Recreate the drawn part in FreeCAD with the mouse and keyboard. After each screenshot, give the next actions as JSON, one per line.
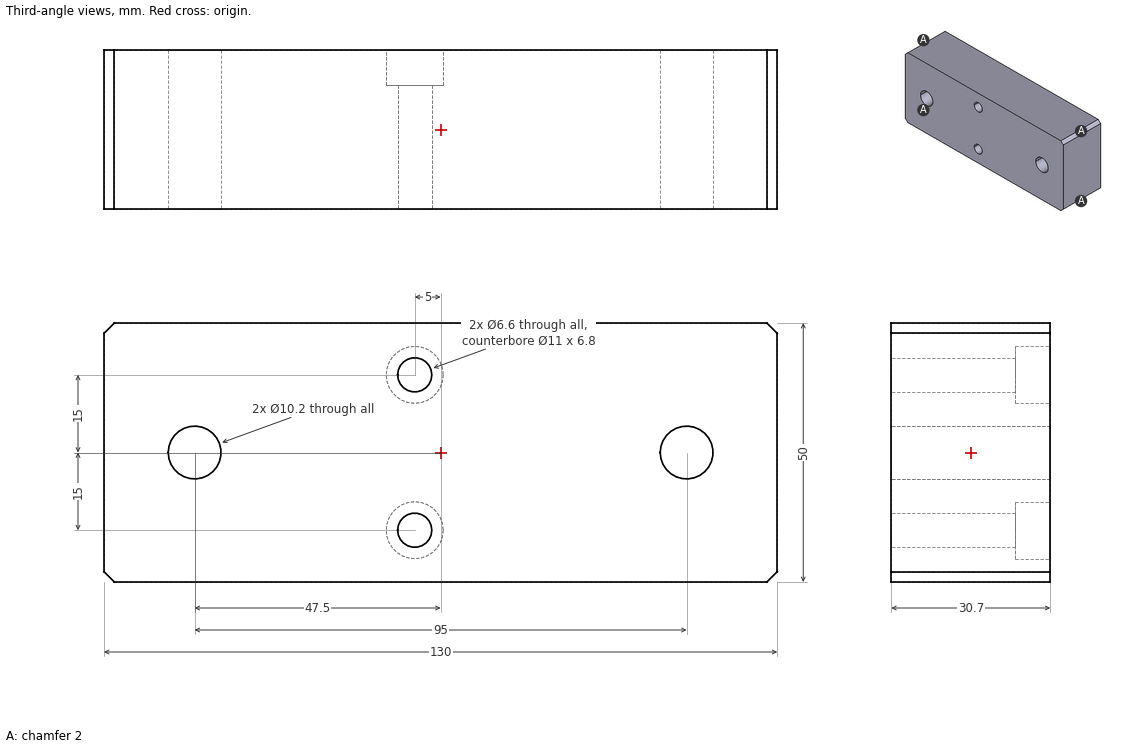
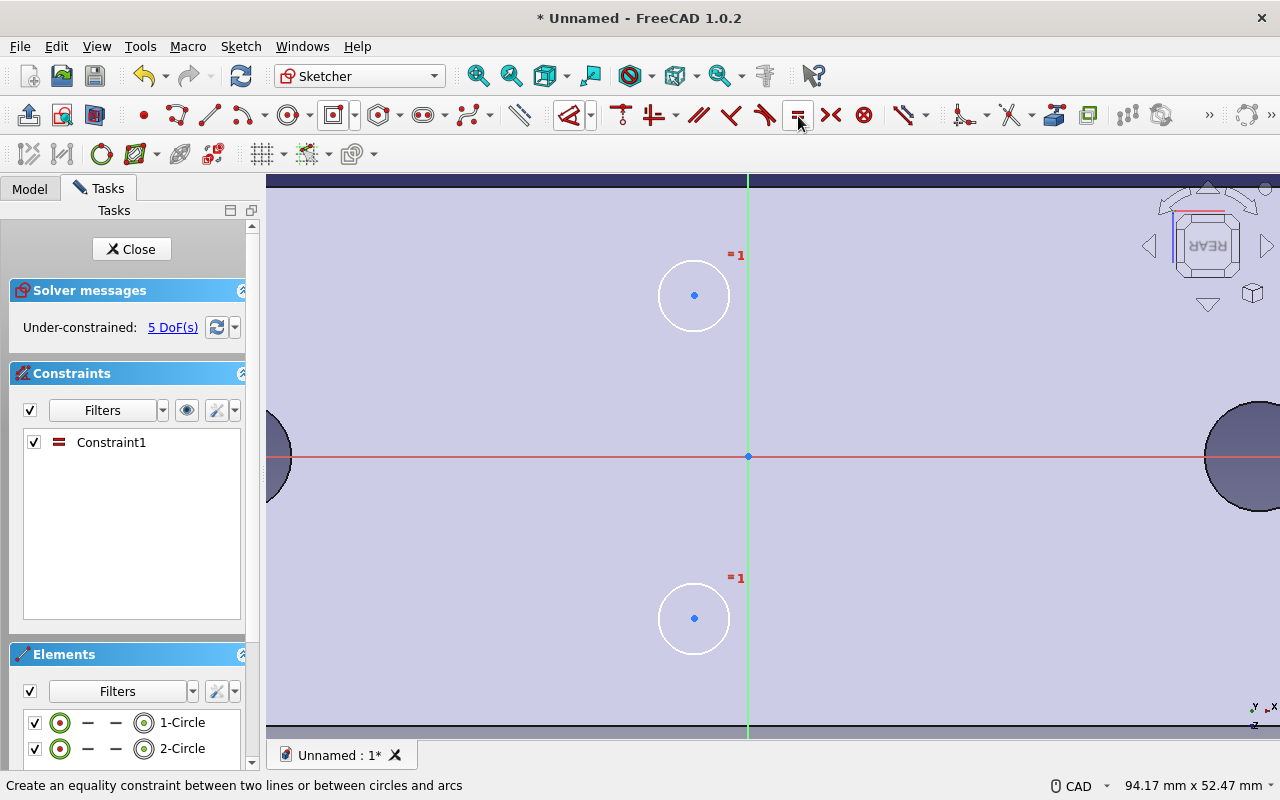
{"action": "left_click", "coordinate": [694, 619]}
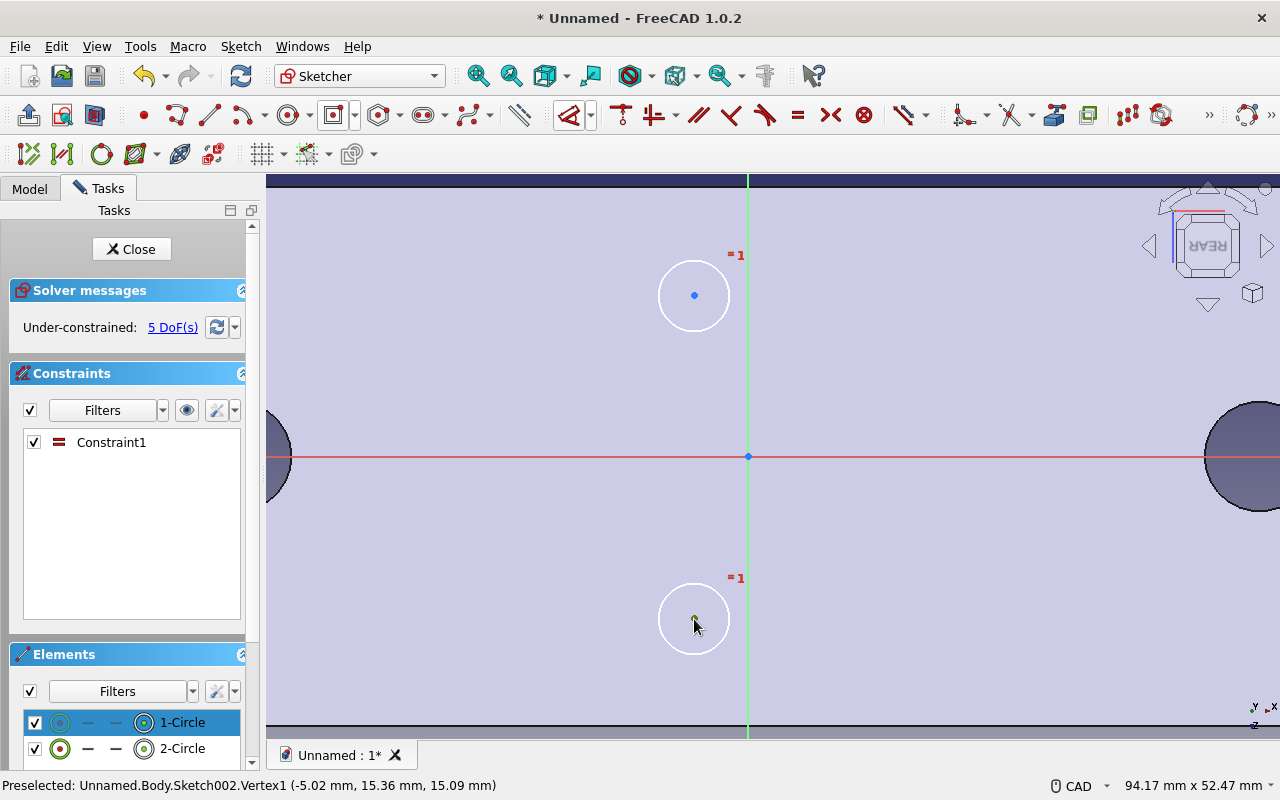
{"action": "left_click", "coordinate": [694, 296]}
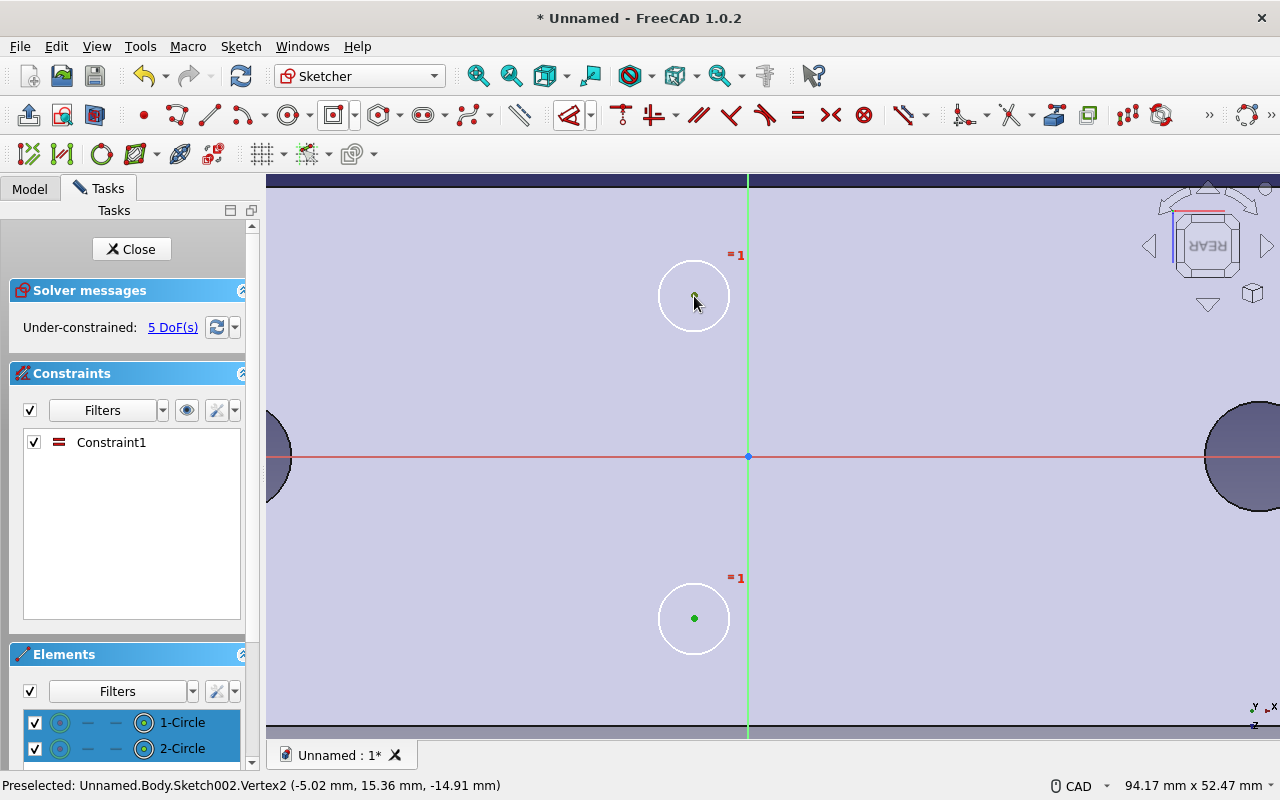
{"action": "left_click", "coordinate": [676, 116]}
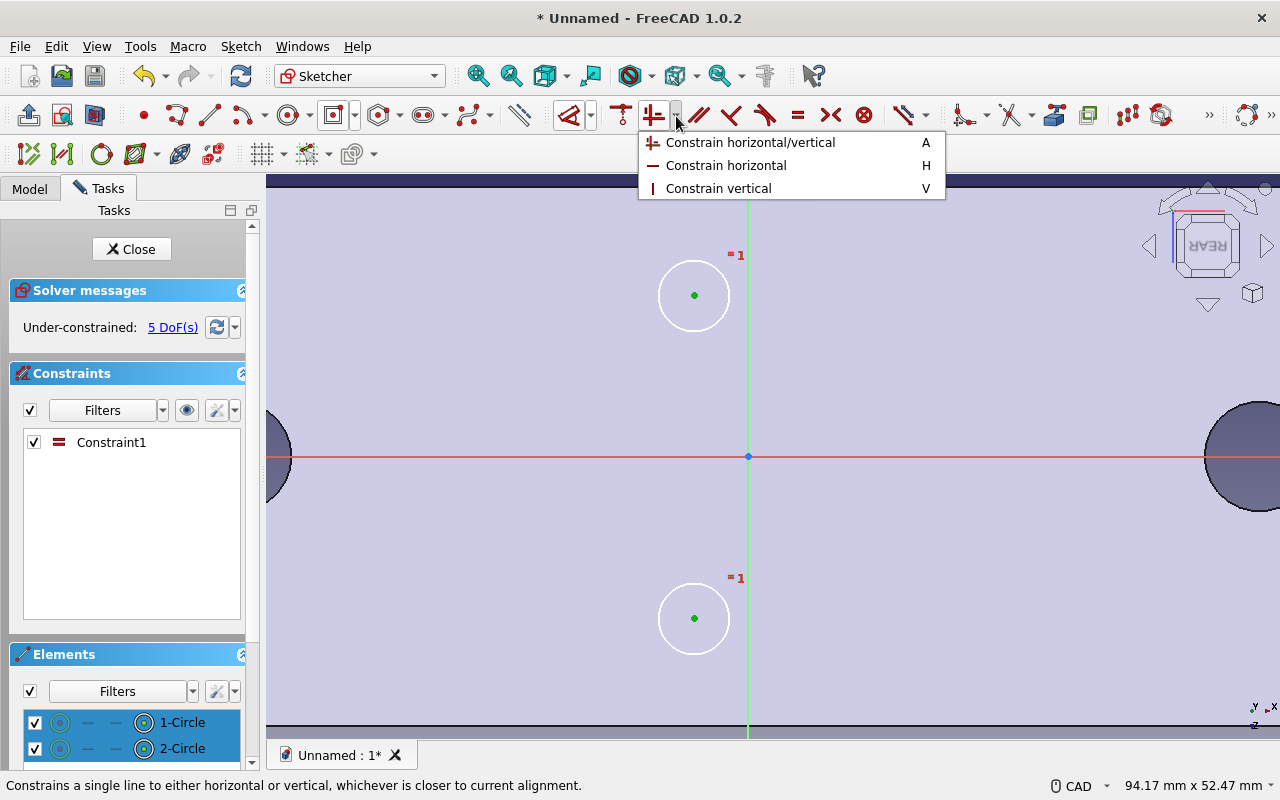
{"action": "left_click", "coordinate": [792, 188]}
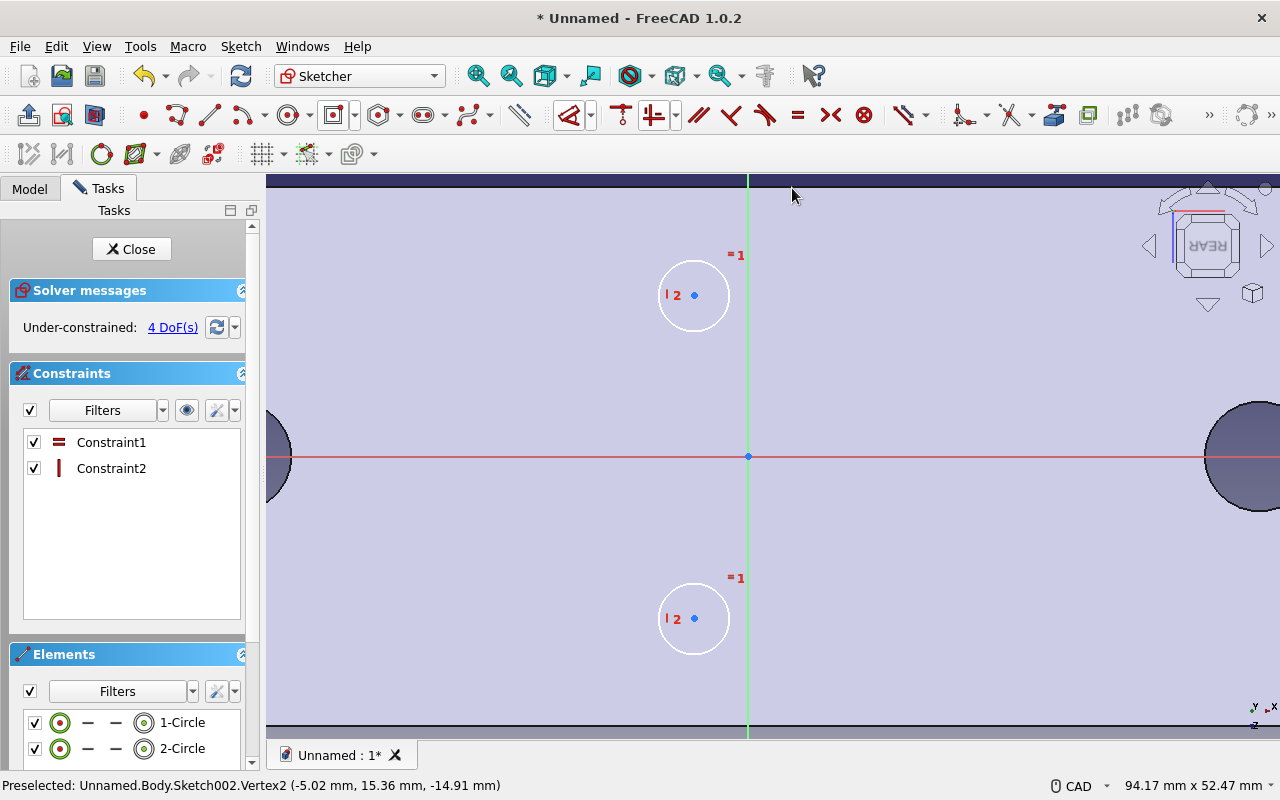
{"action": "left_click", "coordinate": [719, 594]}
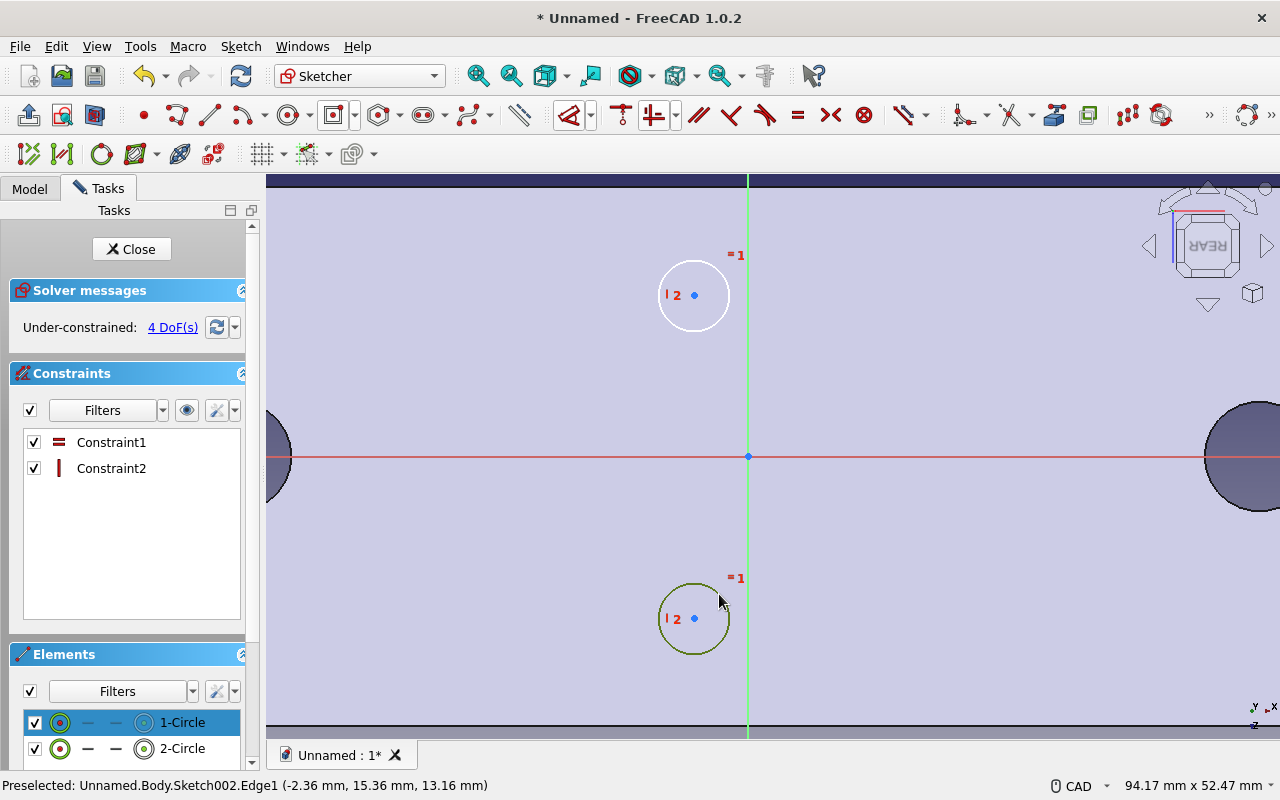
{"action": "left_click", "coordinate": [590, 116]}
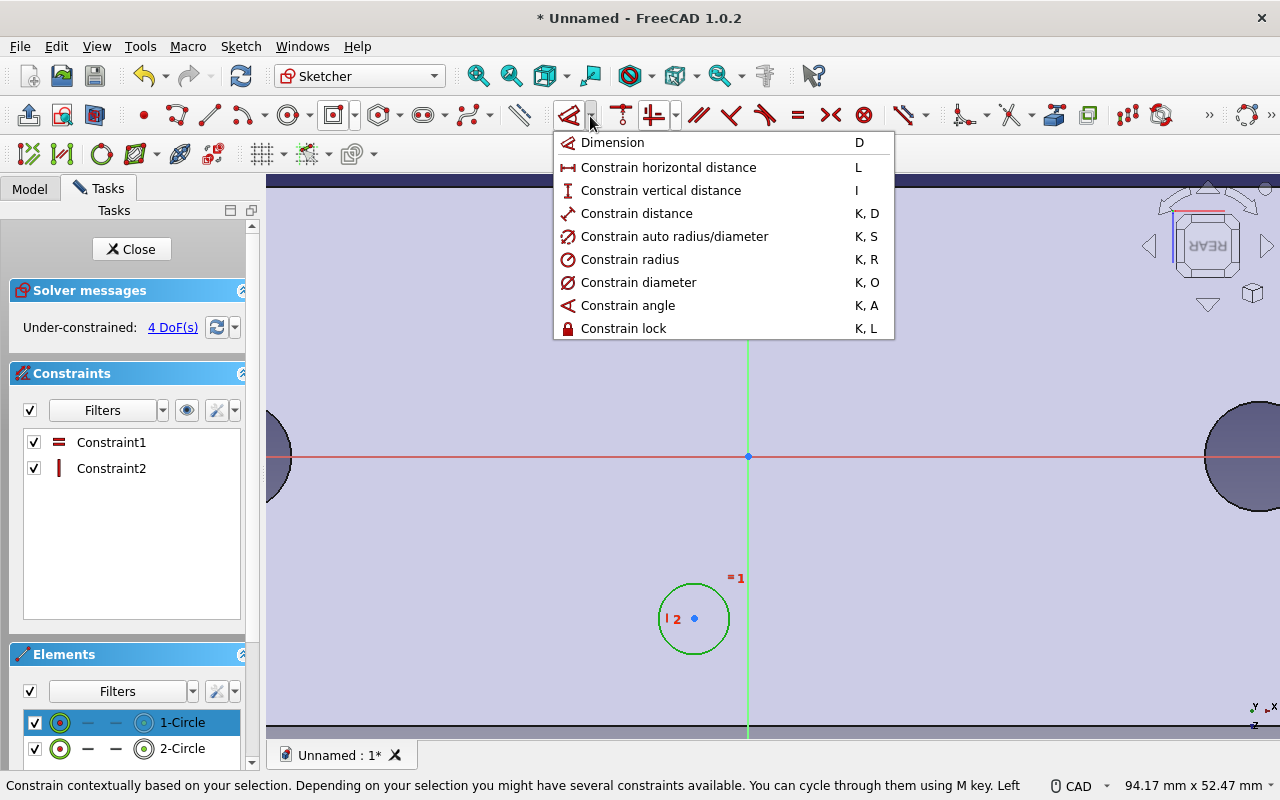
{"action": "left_click", "coordinate": [724, 282]}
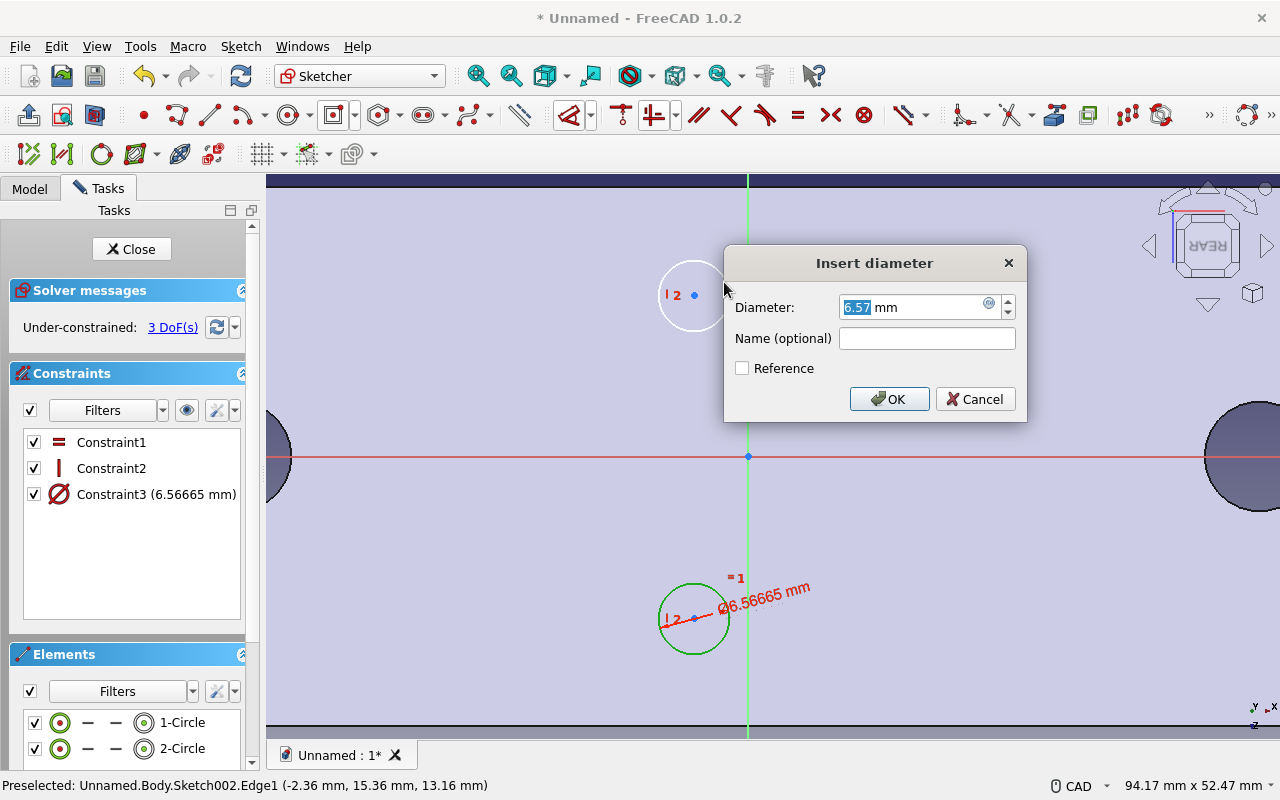
{"action": "type", "text": "6.6"}
{"action": "key", "text": "Return"}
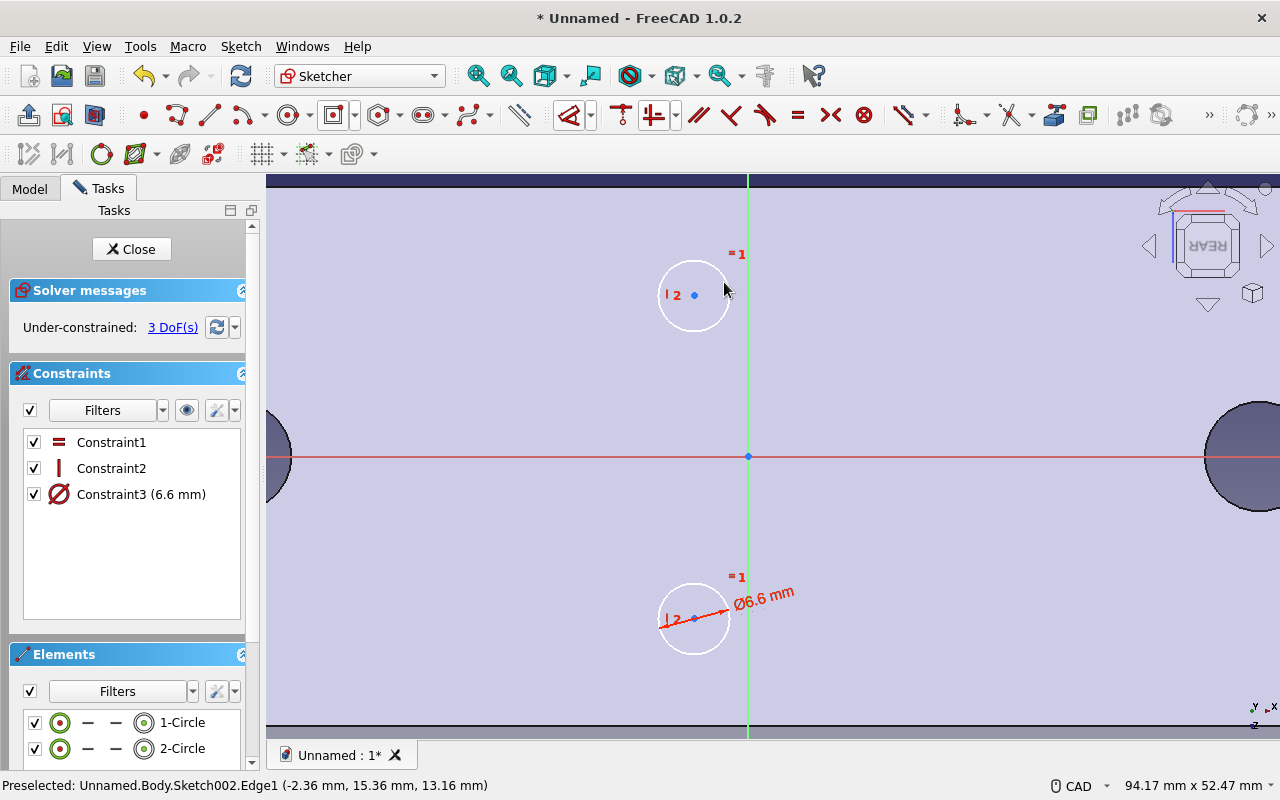
{"action": "left_click", "coordinate": [694, 619]}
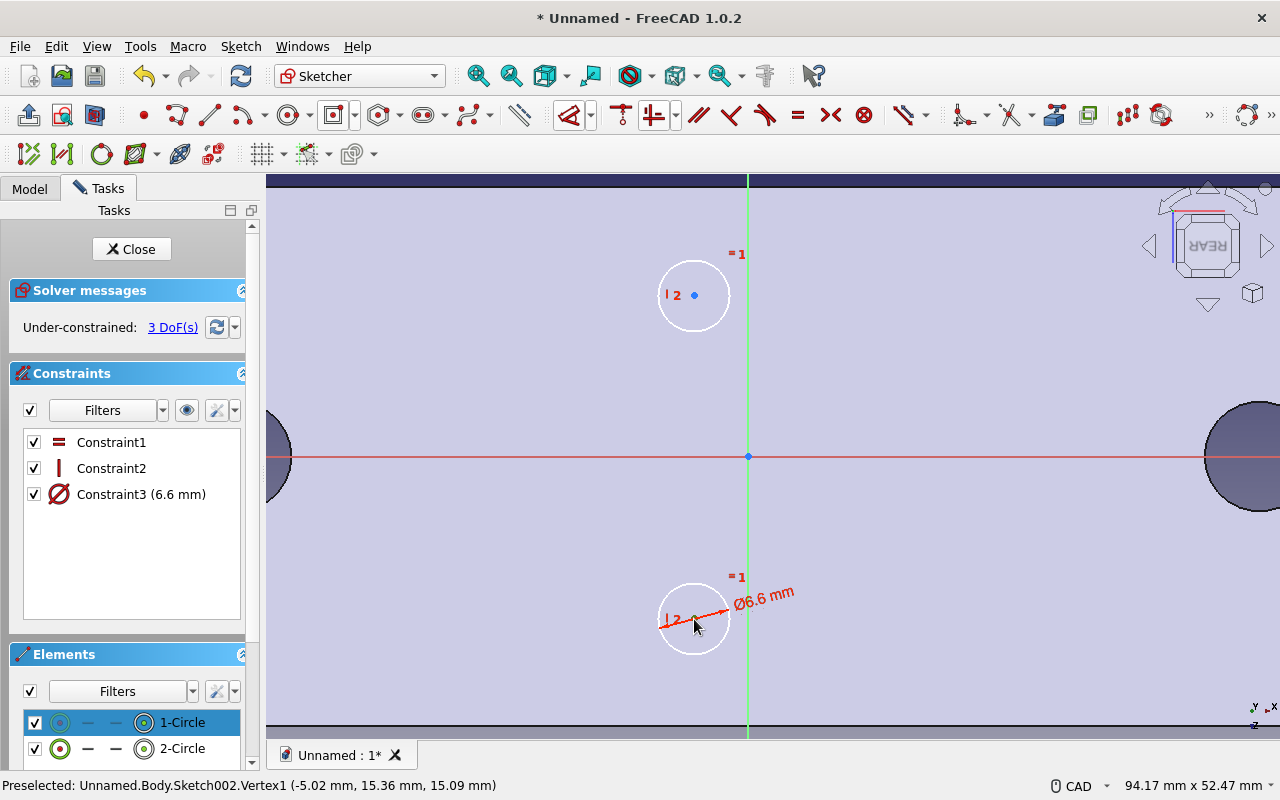
{"action": "left_click", "coordinate": [590, 116]}